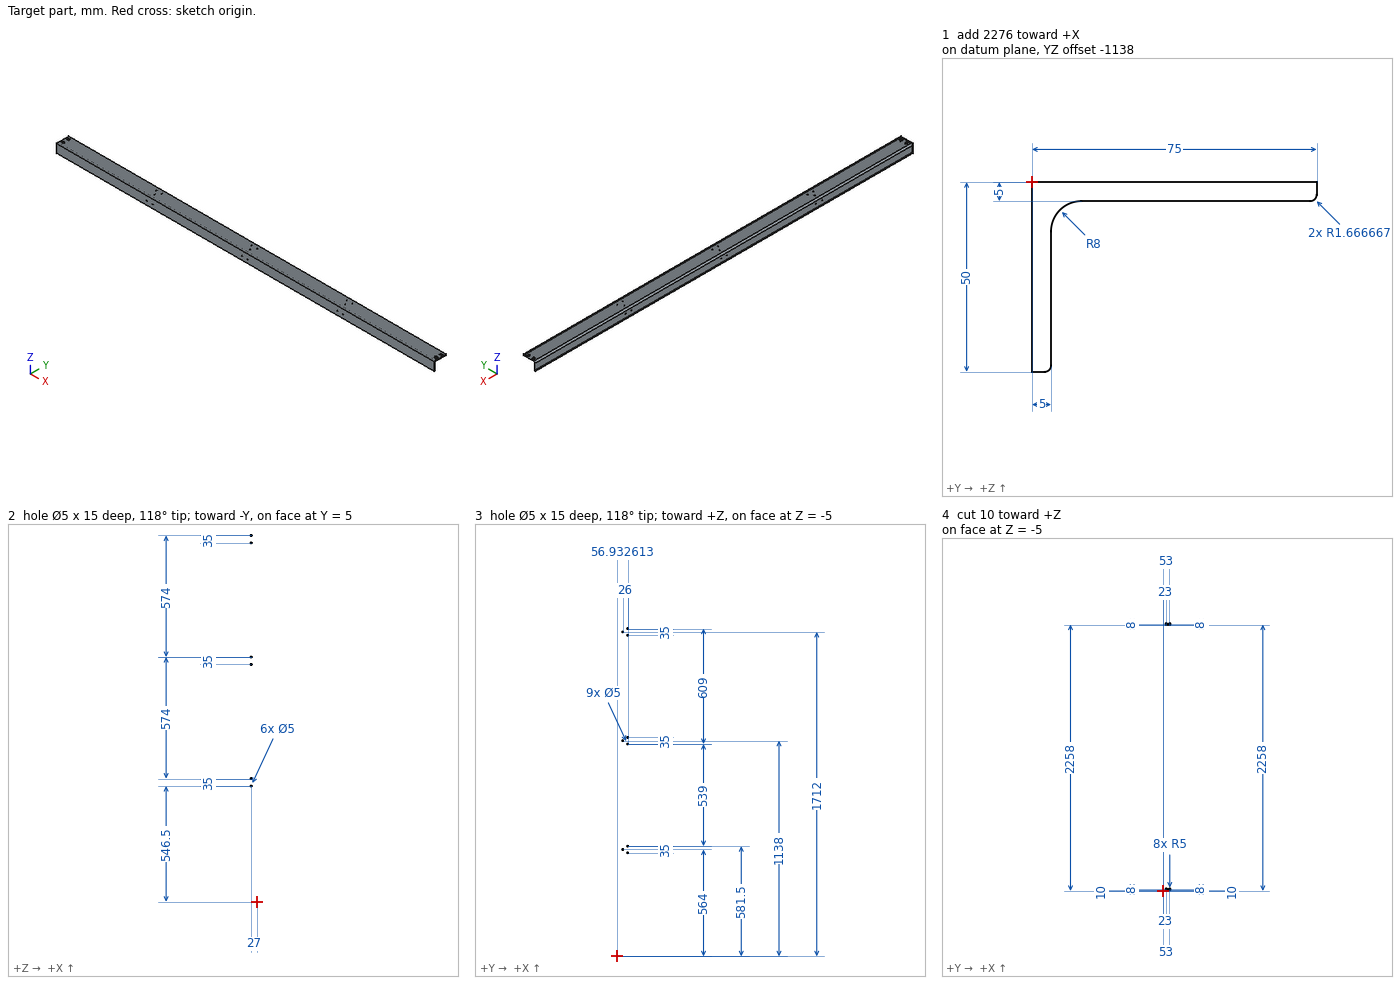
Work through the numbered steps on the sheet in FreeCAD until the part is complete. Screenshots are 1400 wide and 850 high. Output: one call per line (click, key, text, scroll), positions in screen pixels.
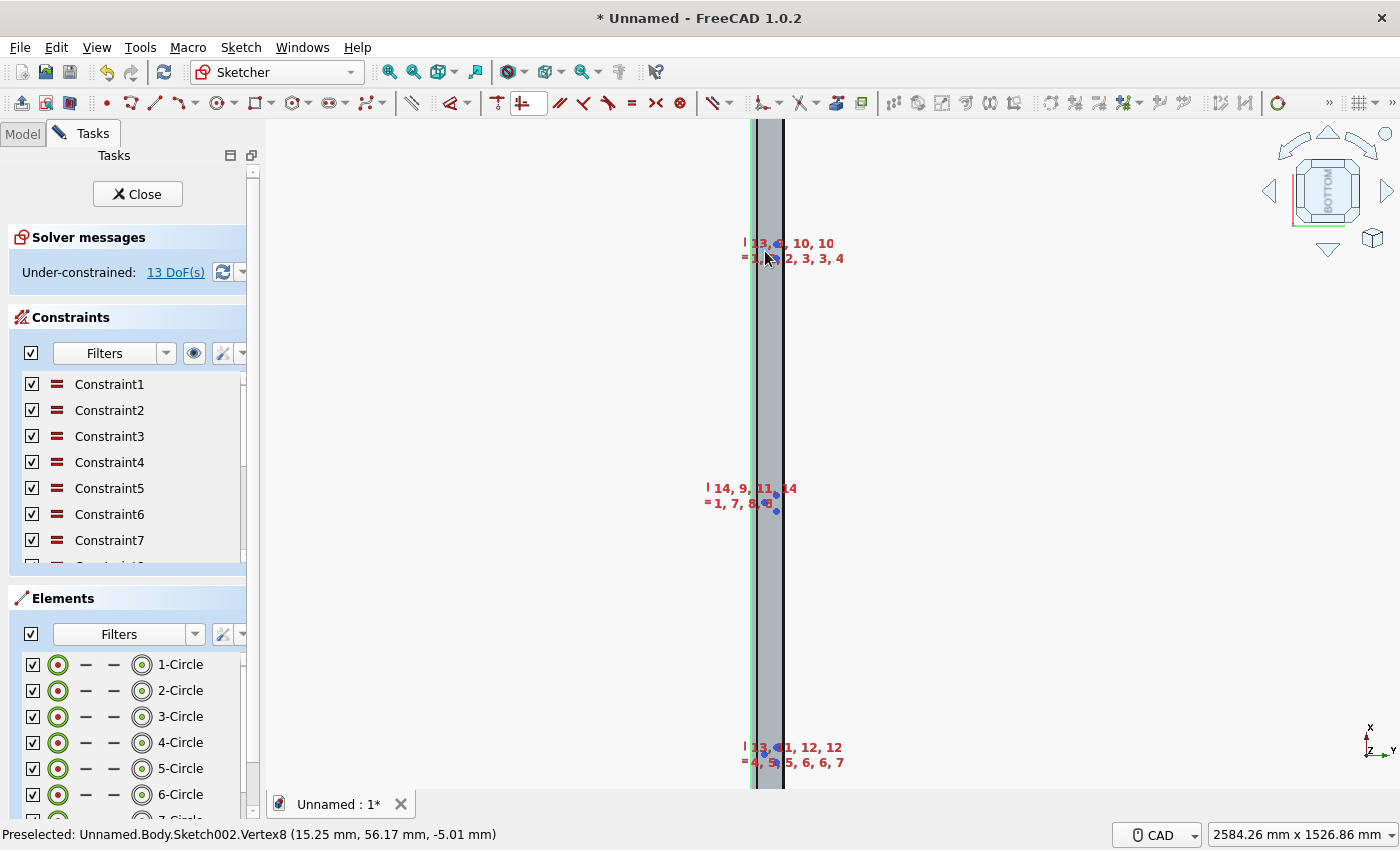
click(765, 250)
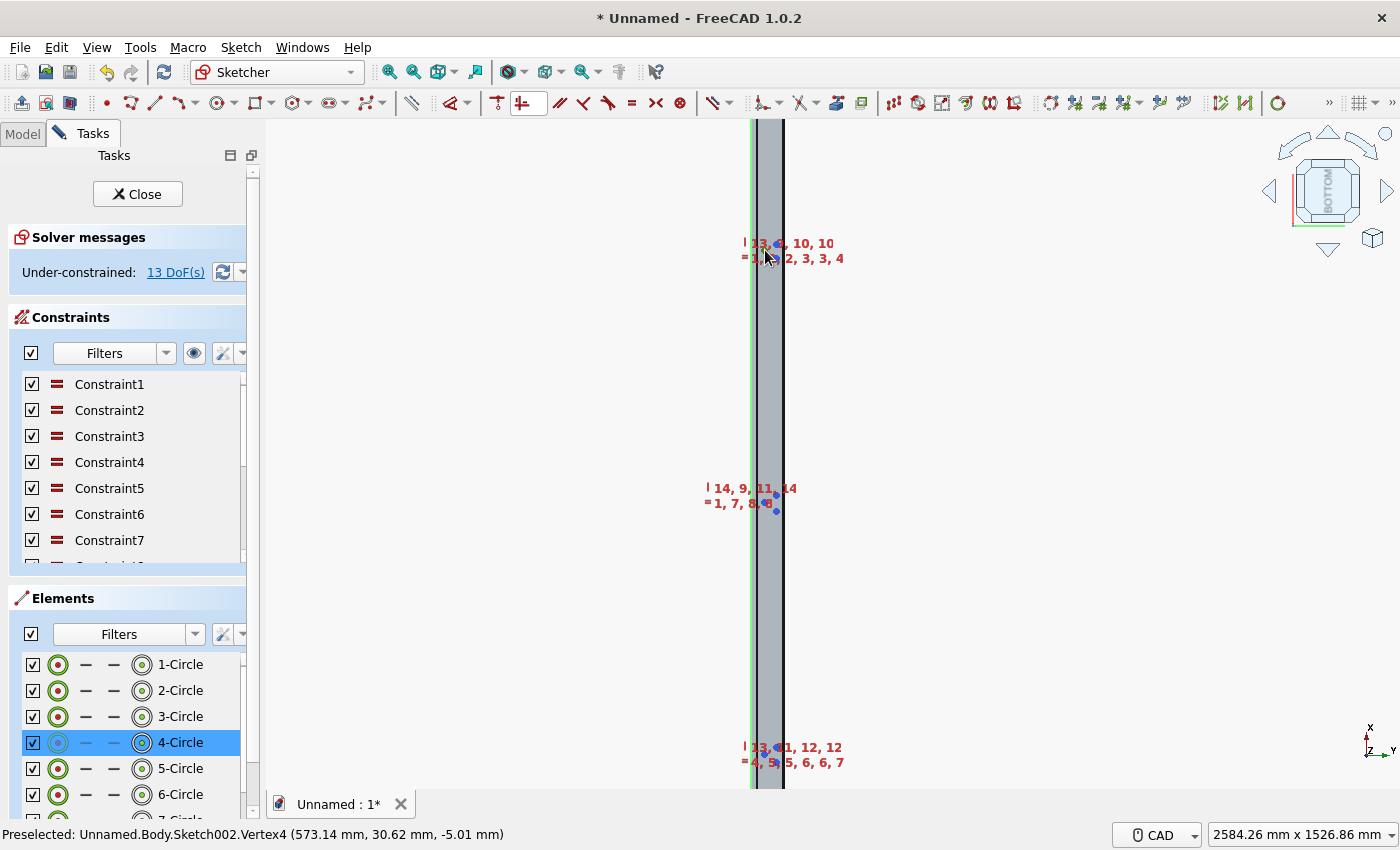
scroll(765, 502, up, 4)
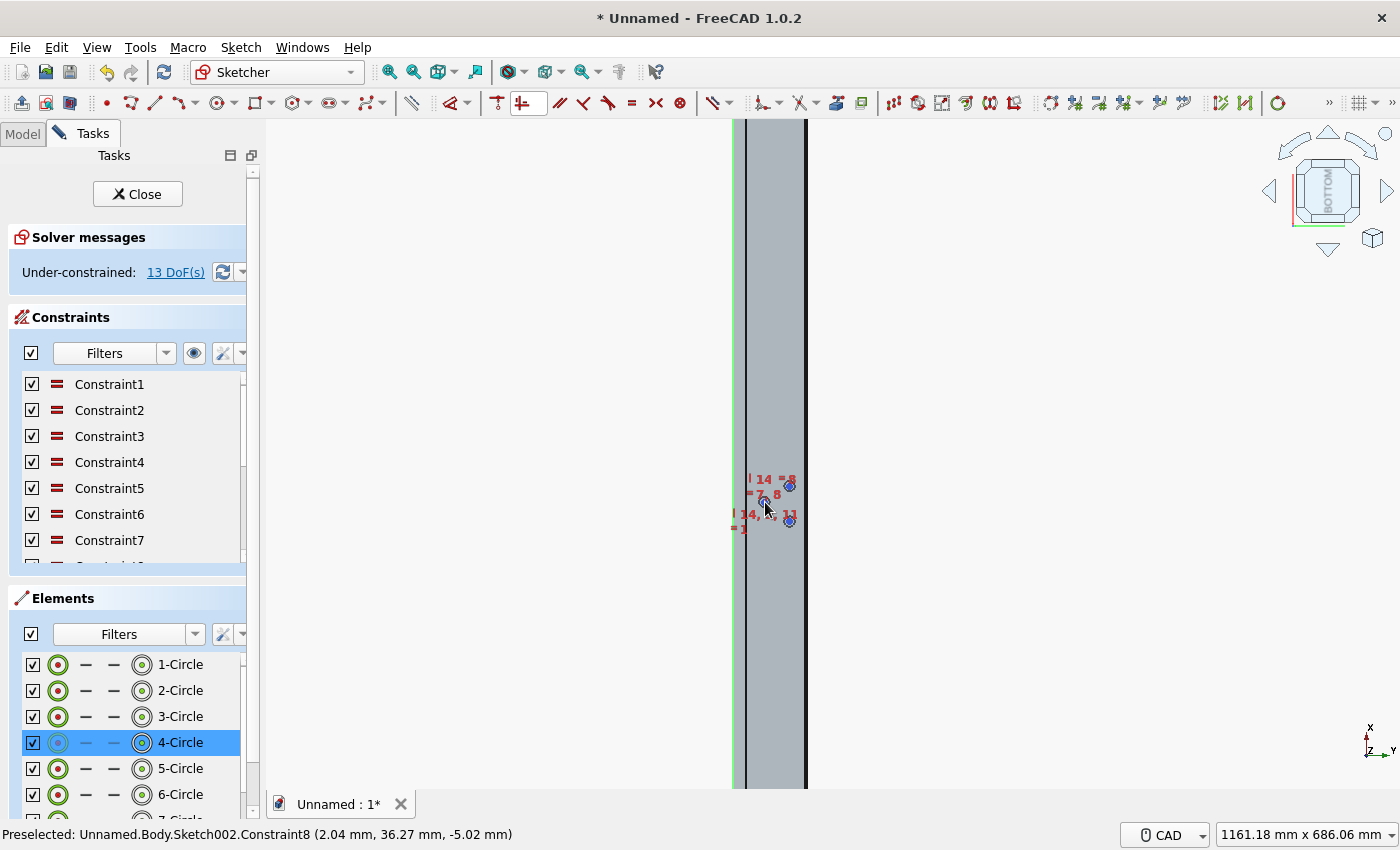
click(764, 502)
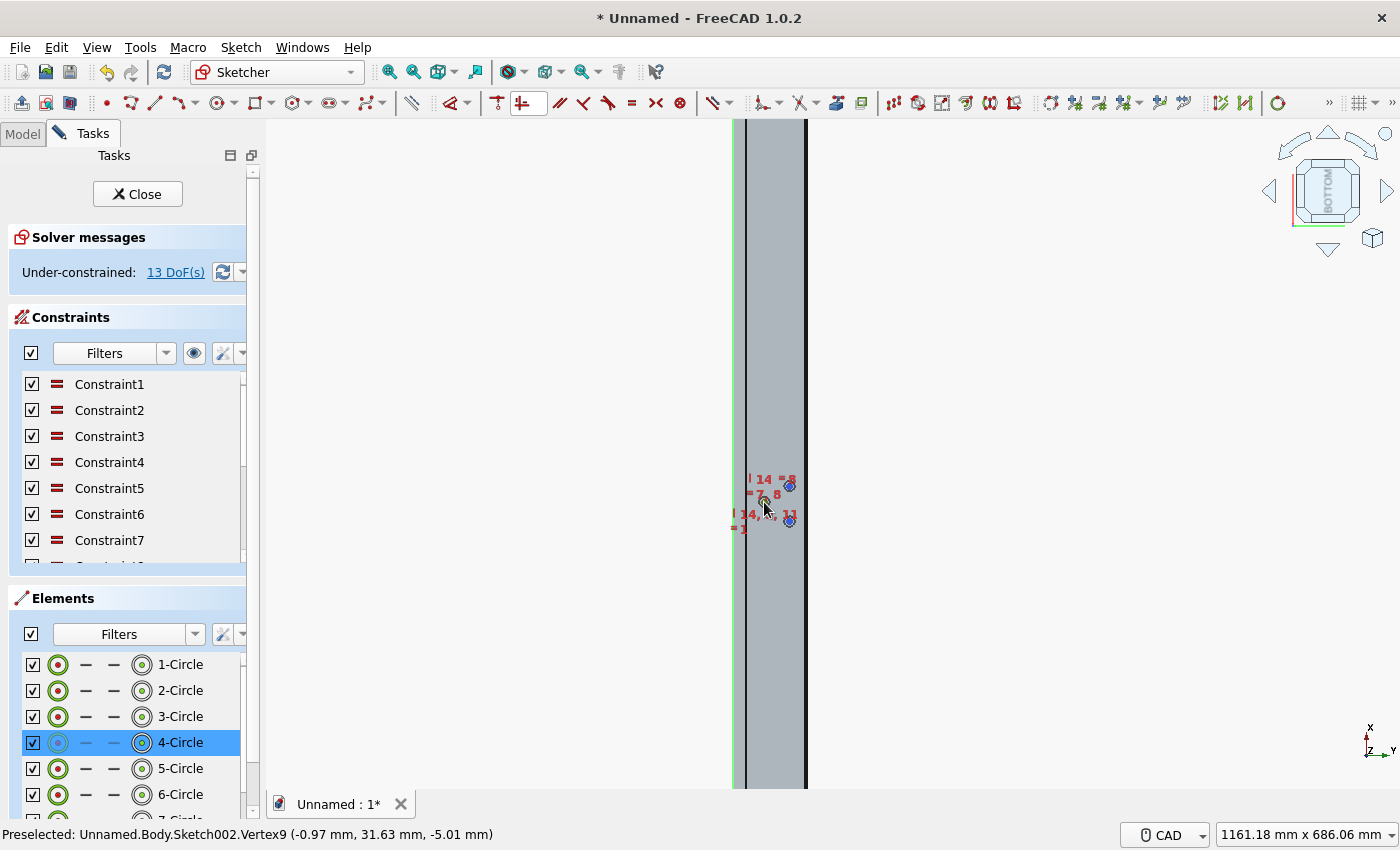
click(542, 104)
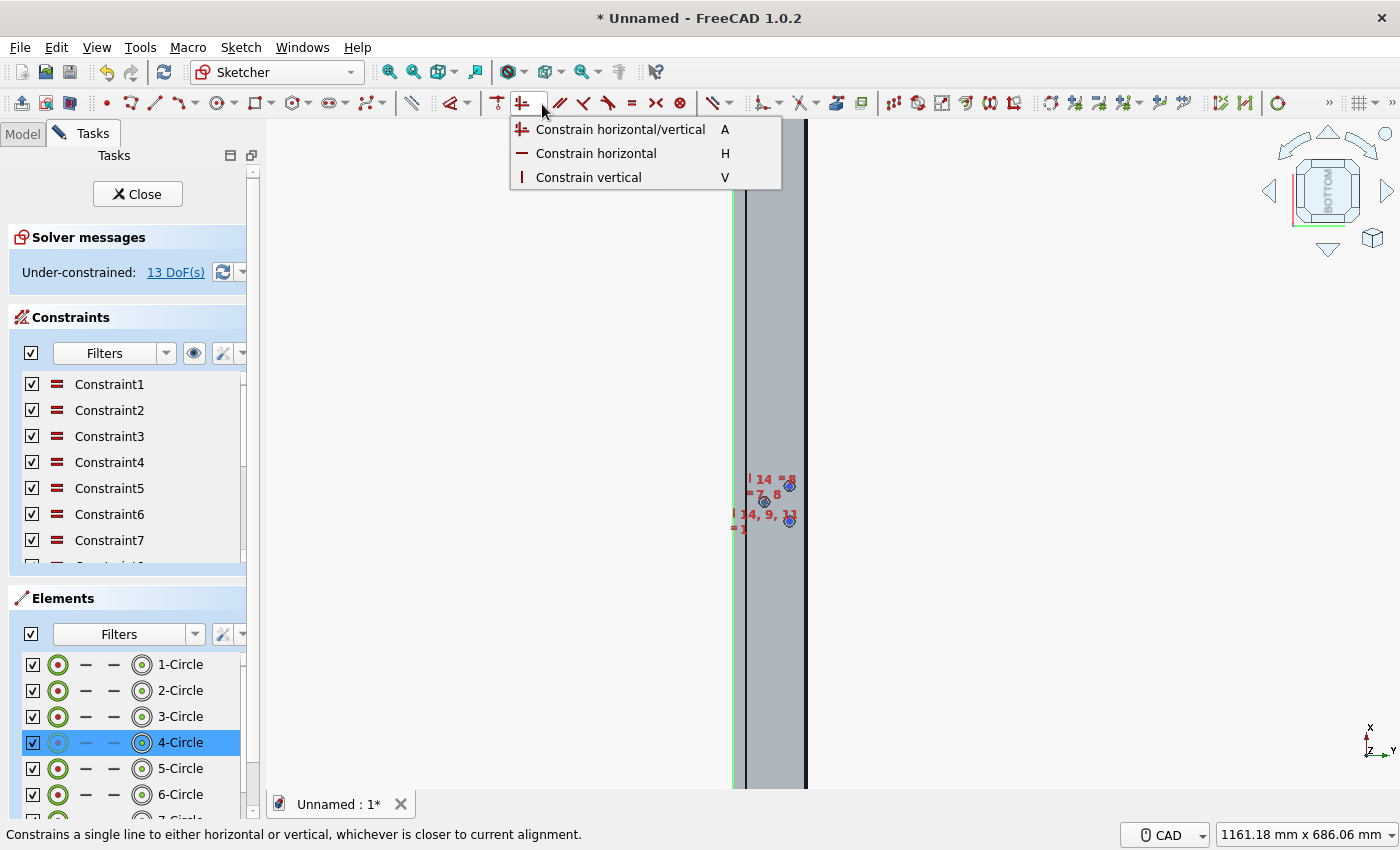
click(646, 177)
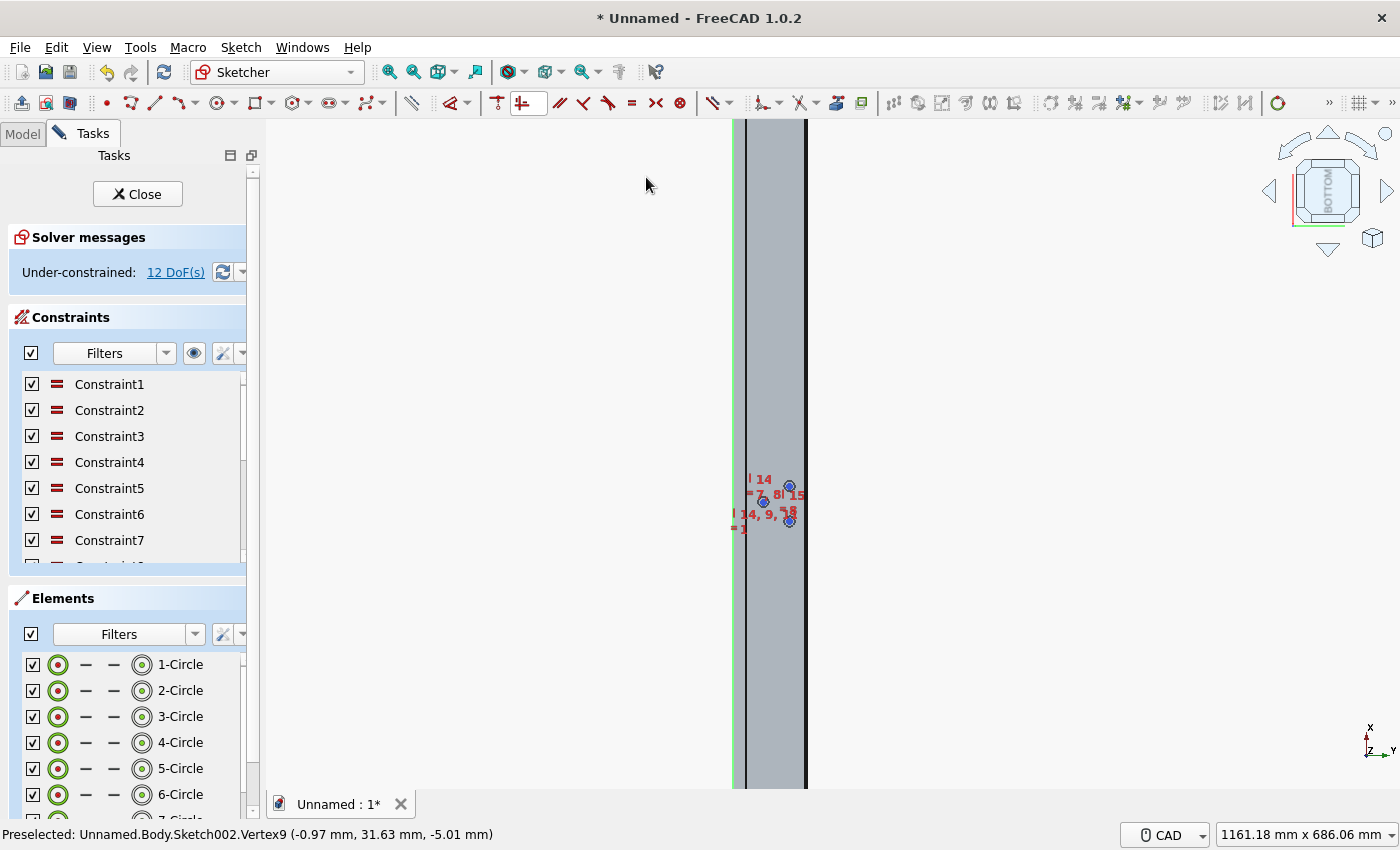
click(450, 104)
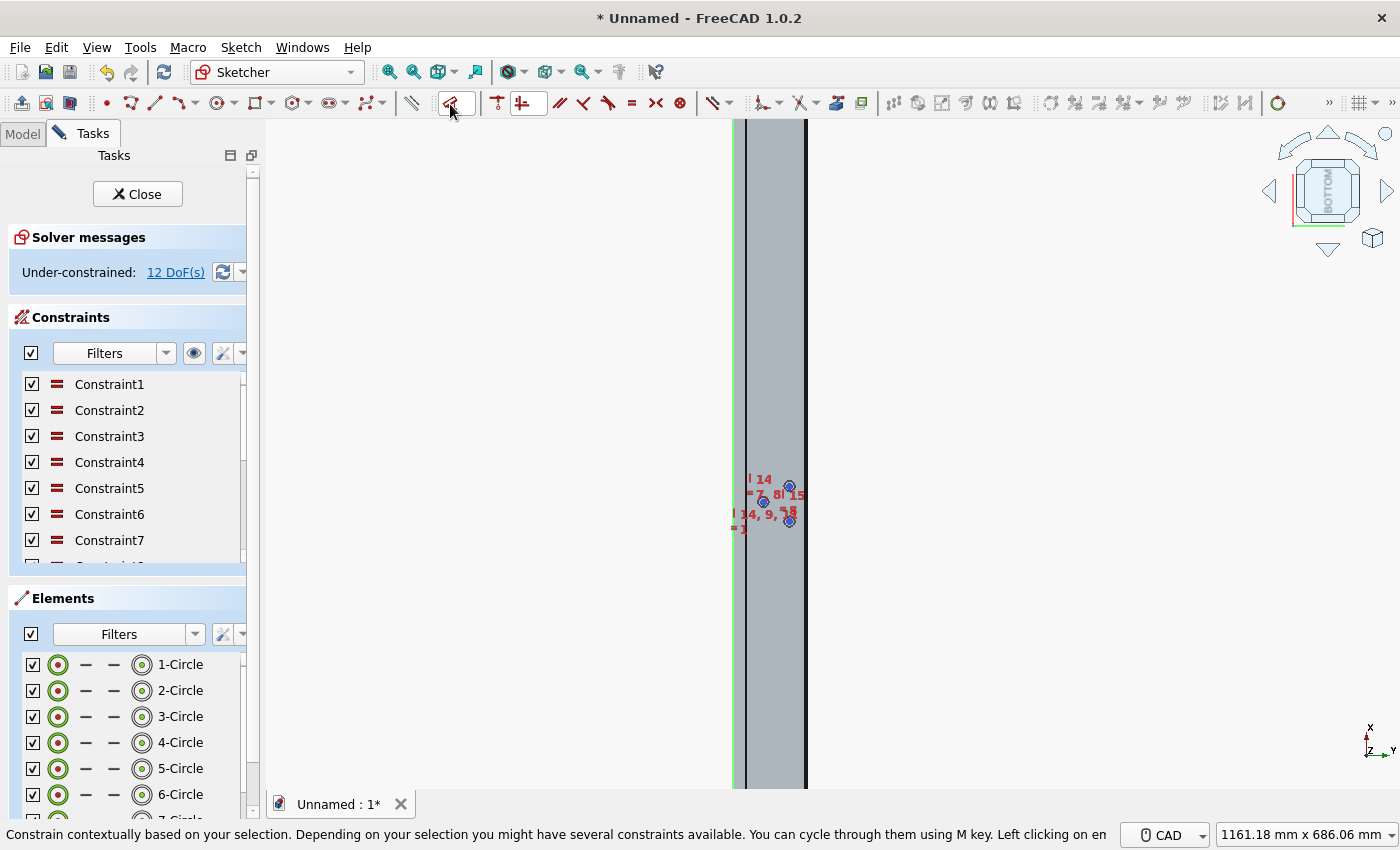
scroll(790, 516, up, 11)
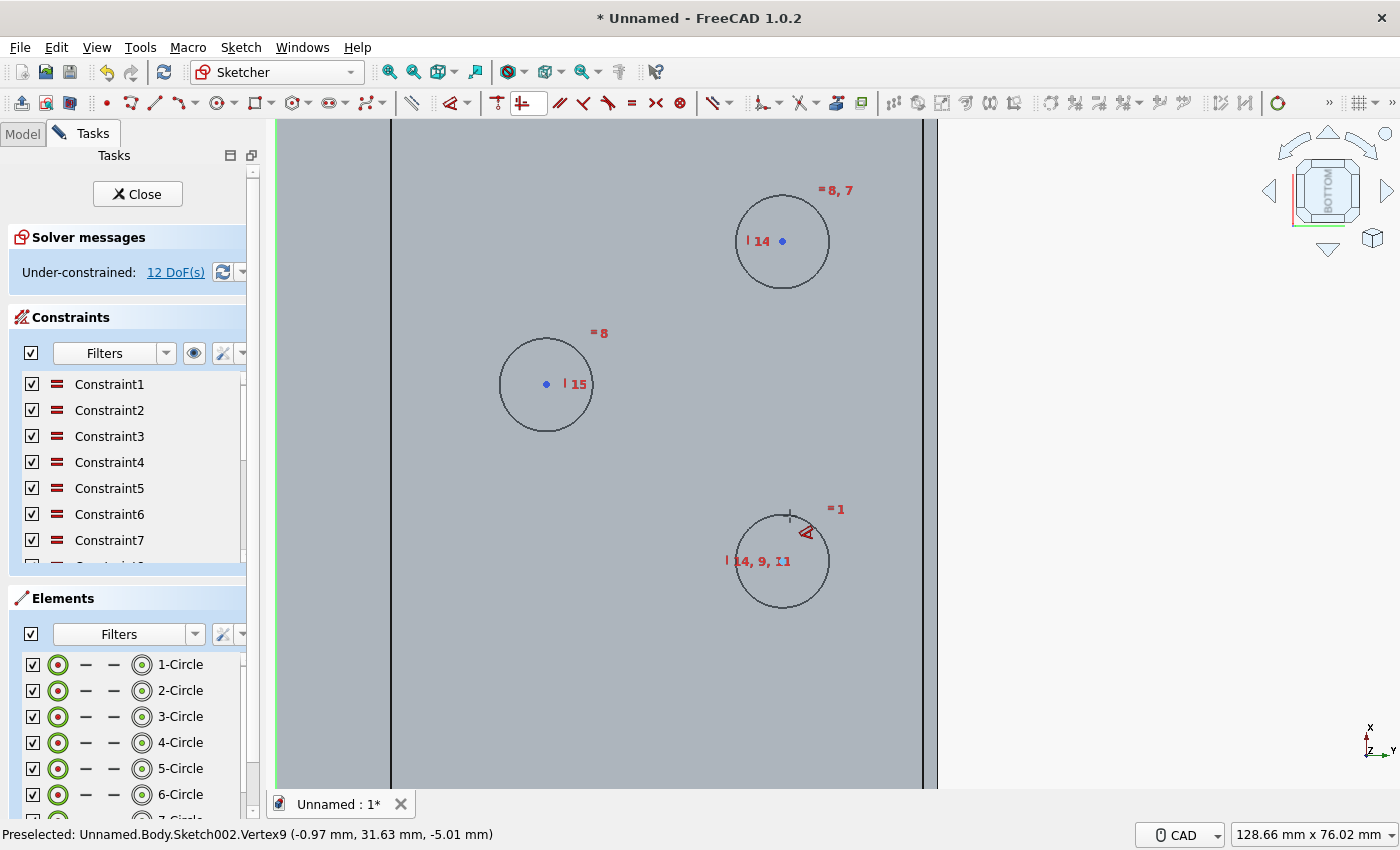
click(784, 515)
click(785, 483)